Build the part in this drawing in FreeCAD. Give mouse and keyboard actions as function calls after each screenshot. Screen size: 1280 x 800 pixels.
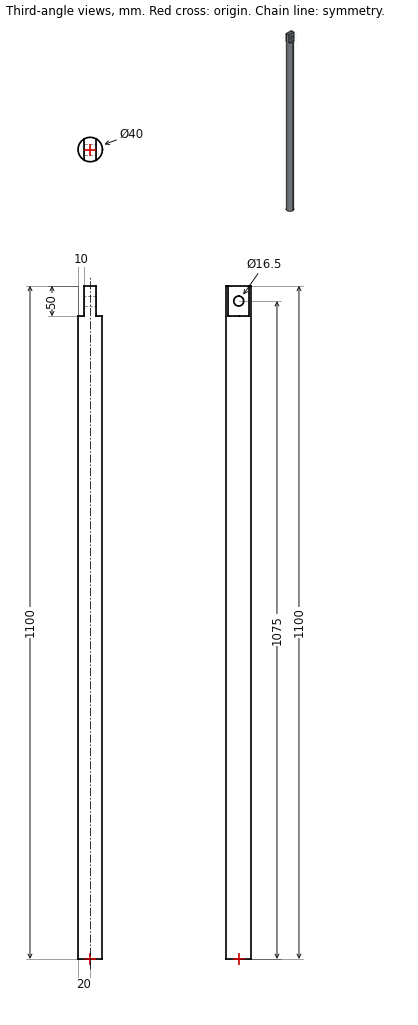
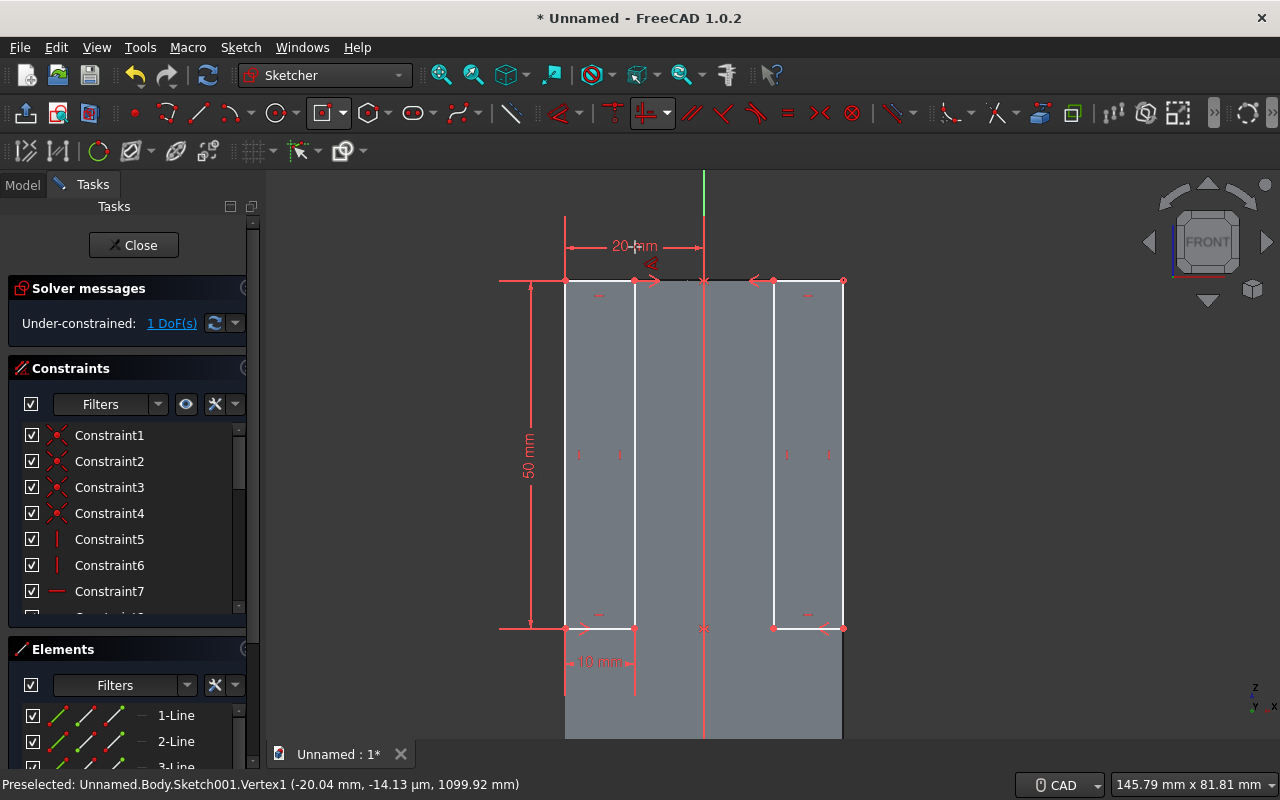
click(565, 281)
click(531, 496)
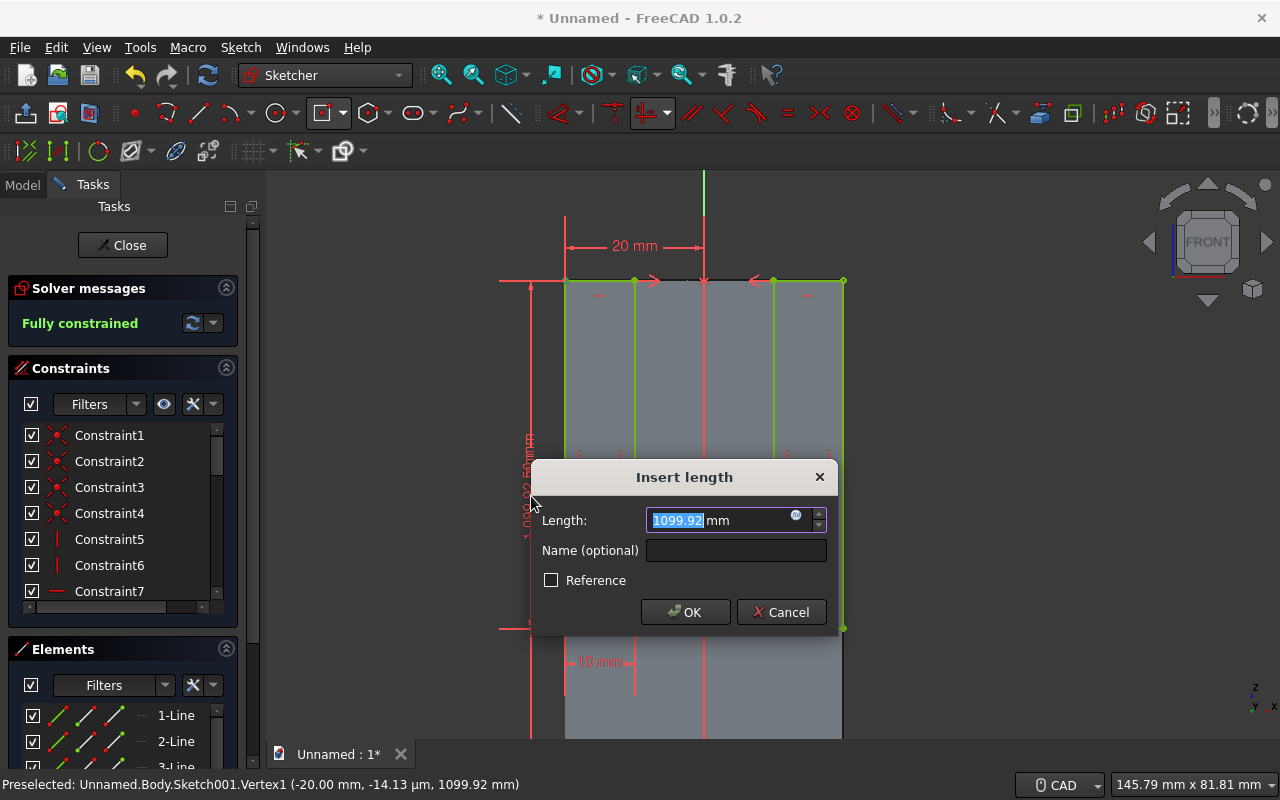
text(1100)
key(Return)
key(Escape)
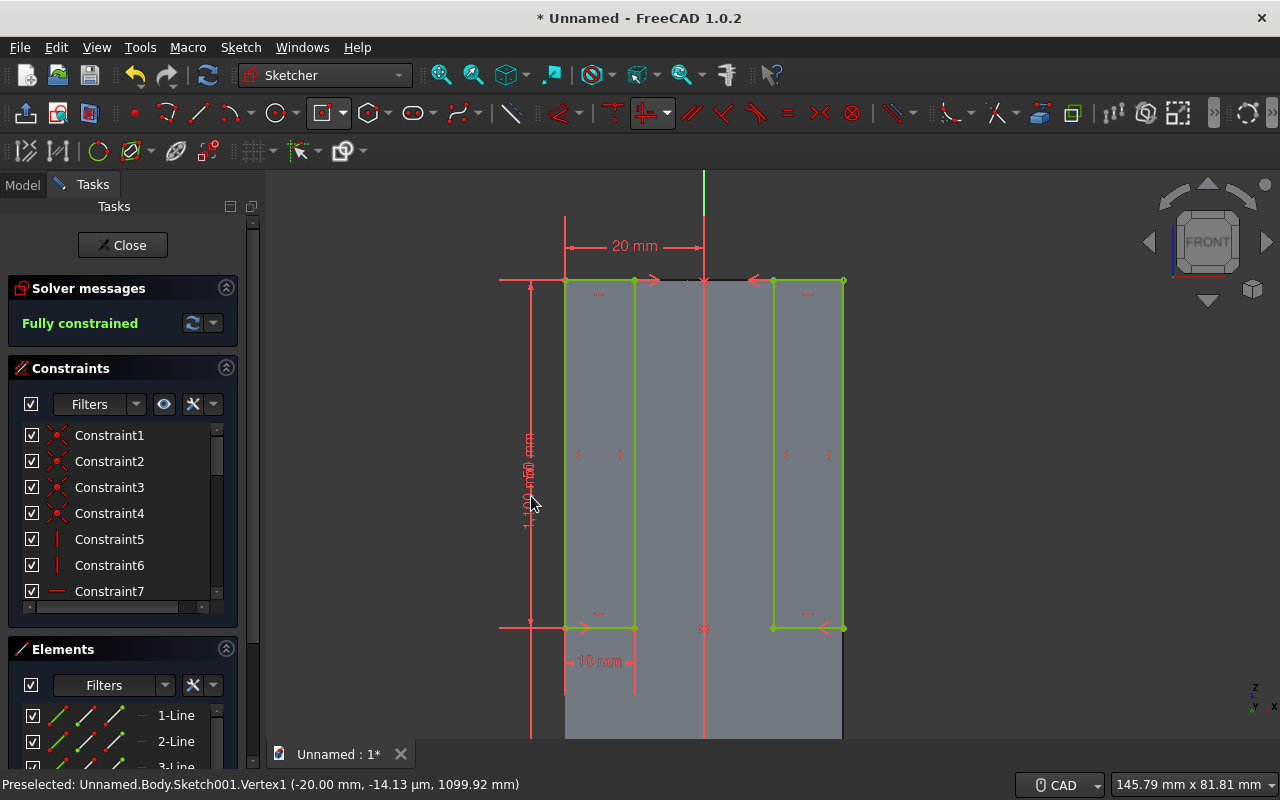
click(123, 245)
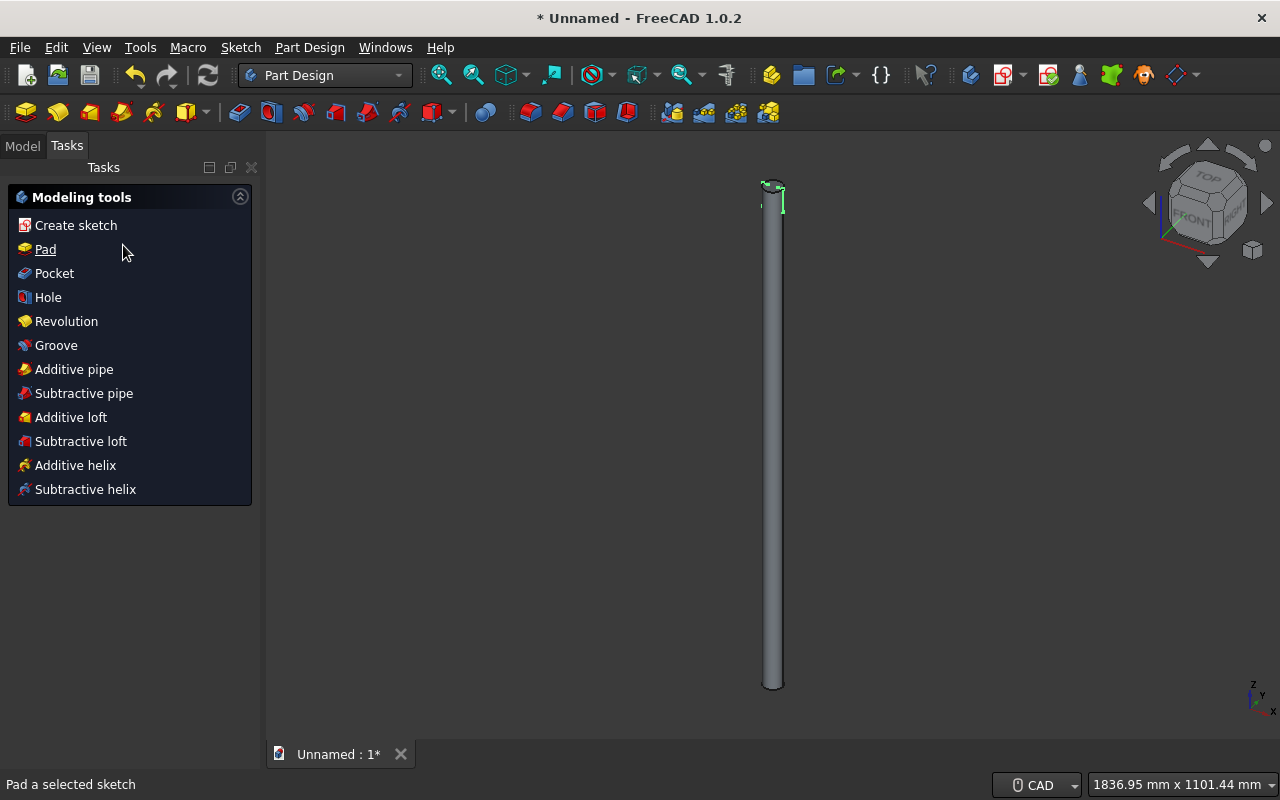
click(240, 112)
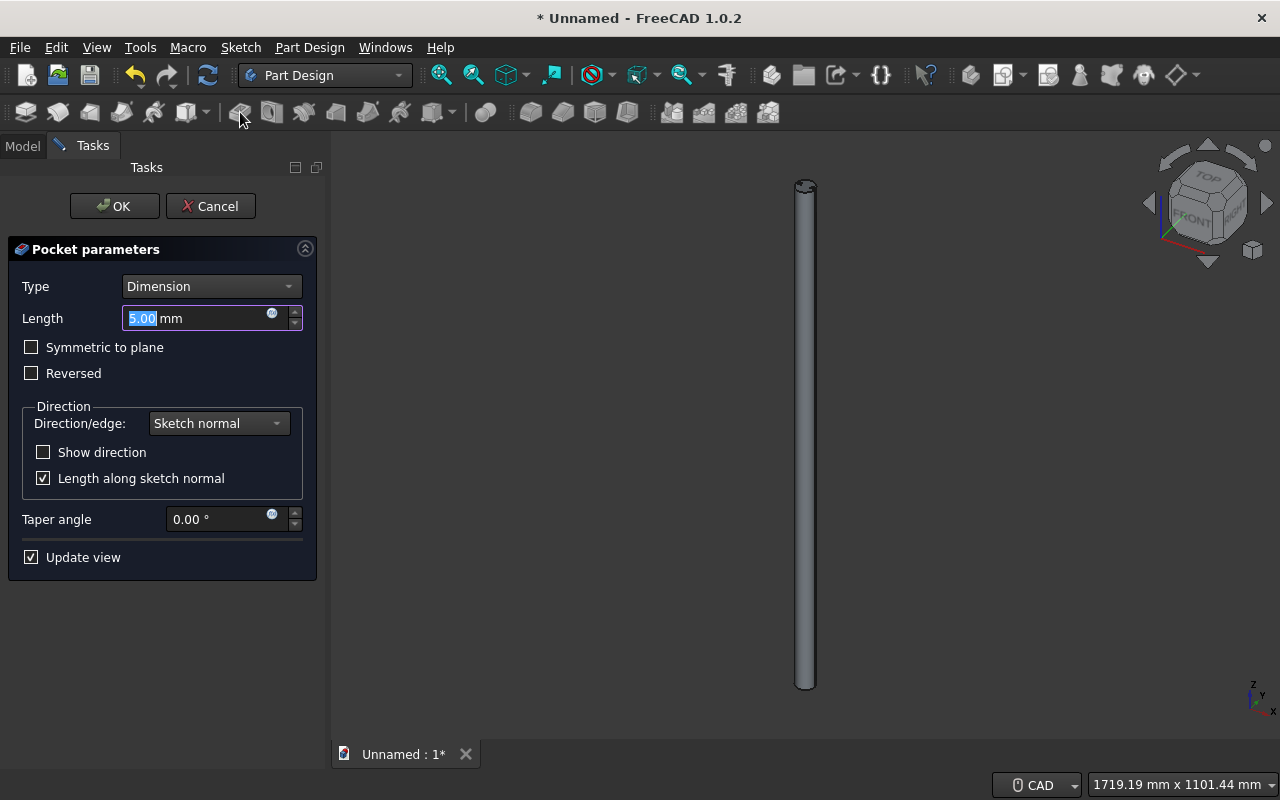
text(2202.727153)
key(Tab)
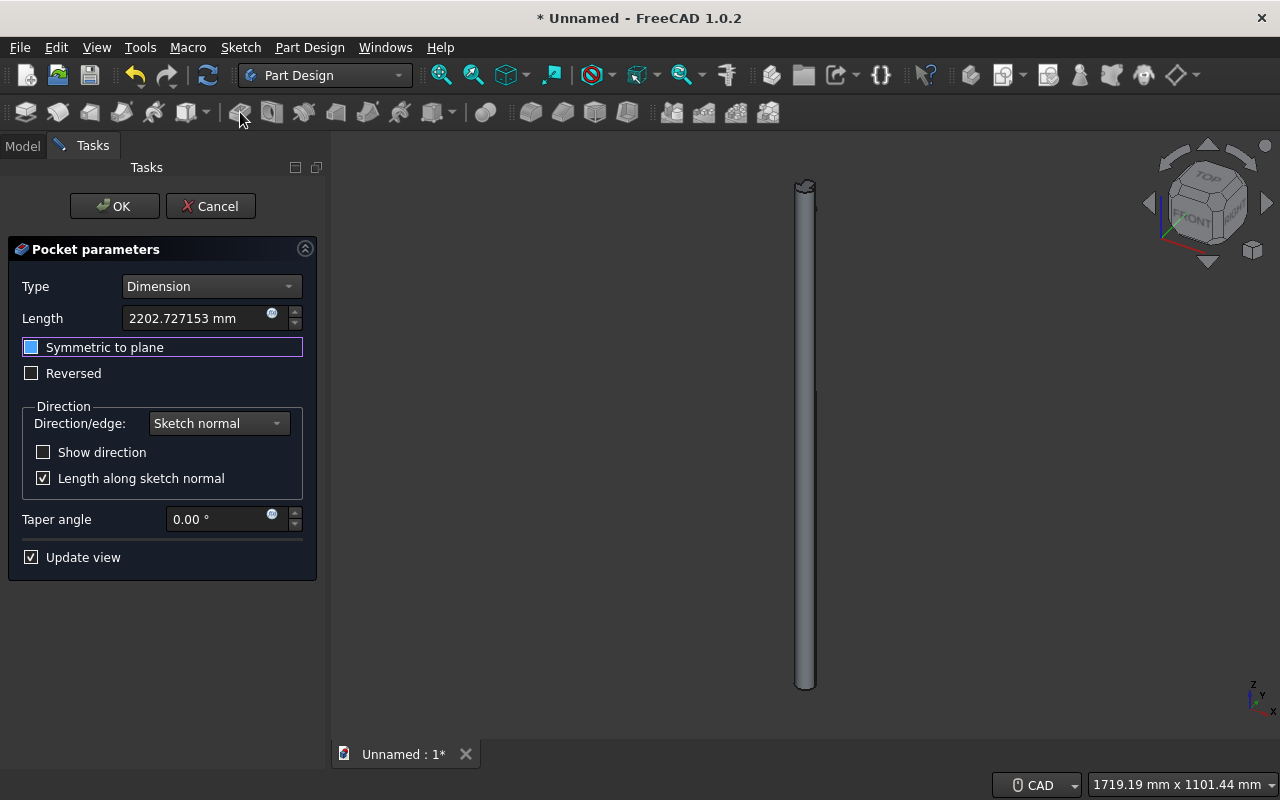
click(30, 347)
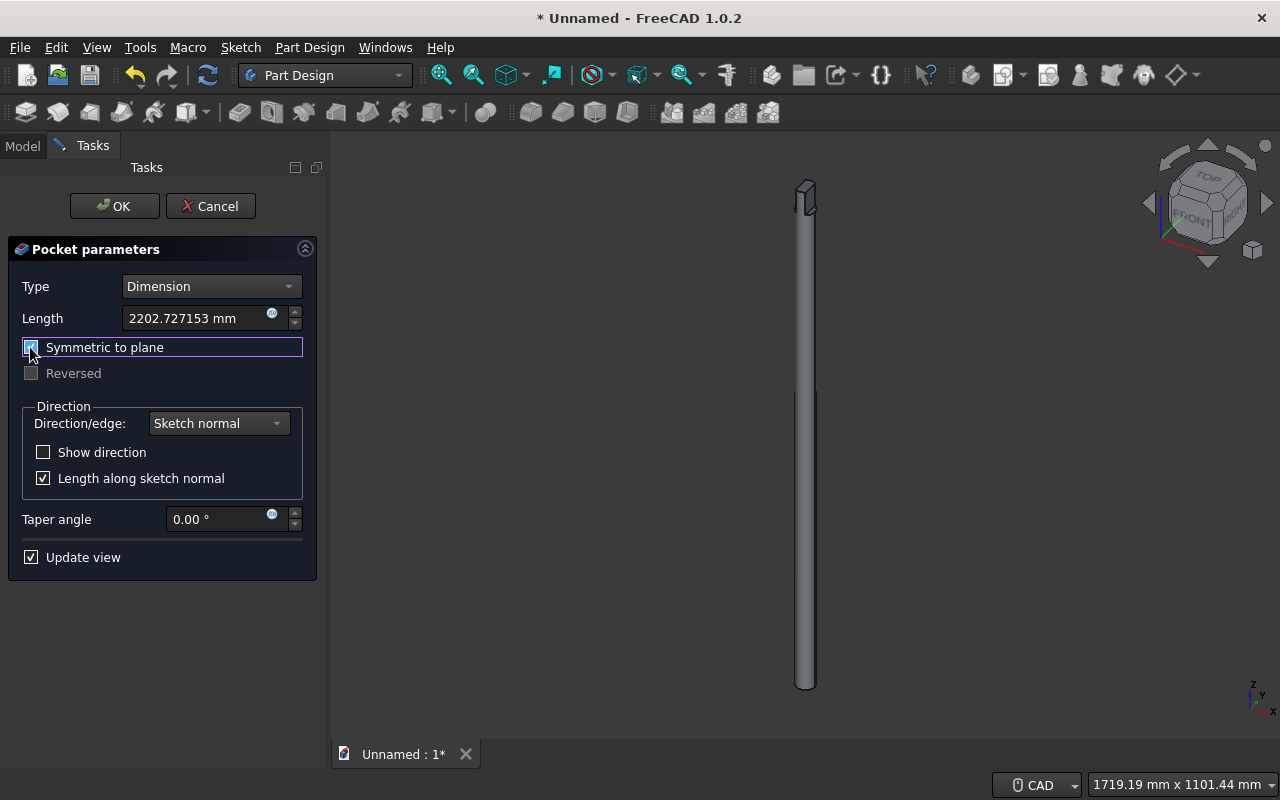
click(115, 206)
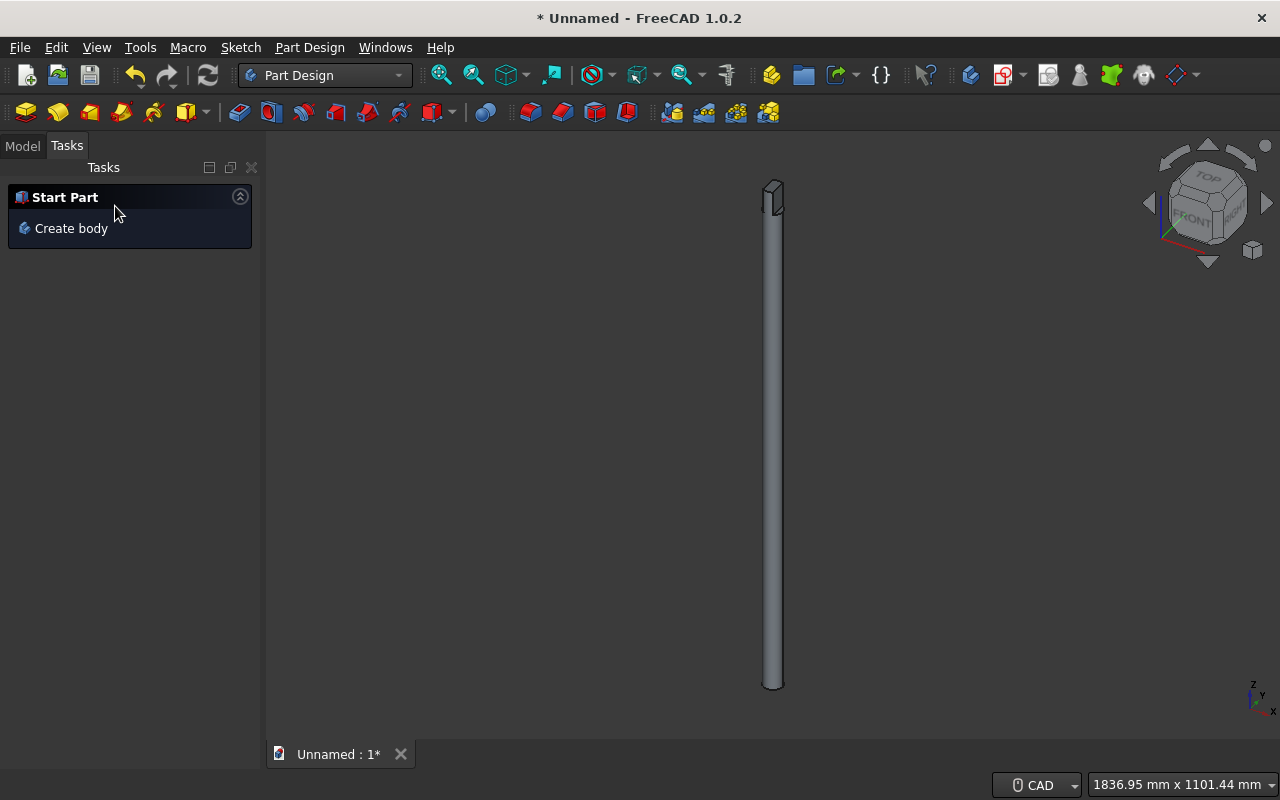
key(6)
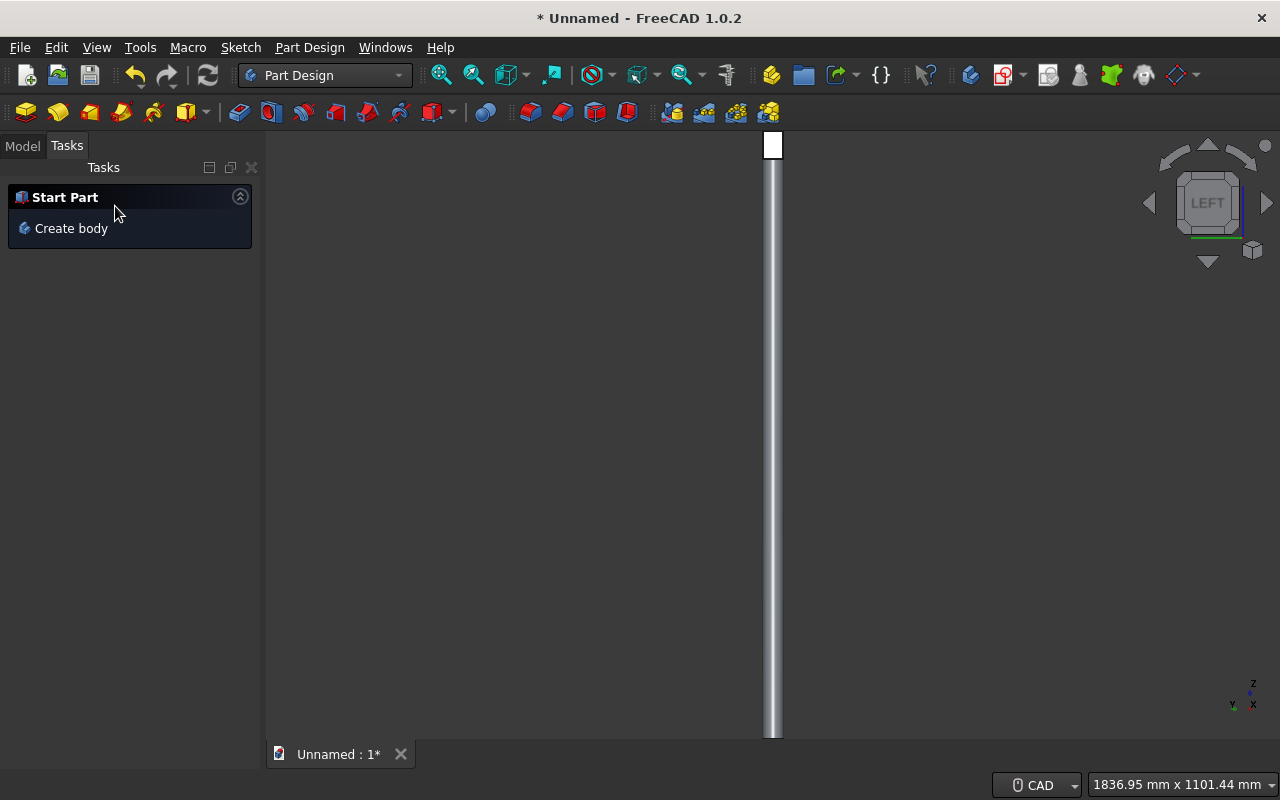
click(442, 76)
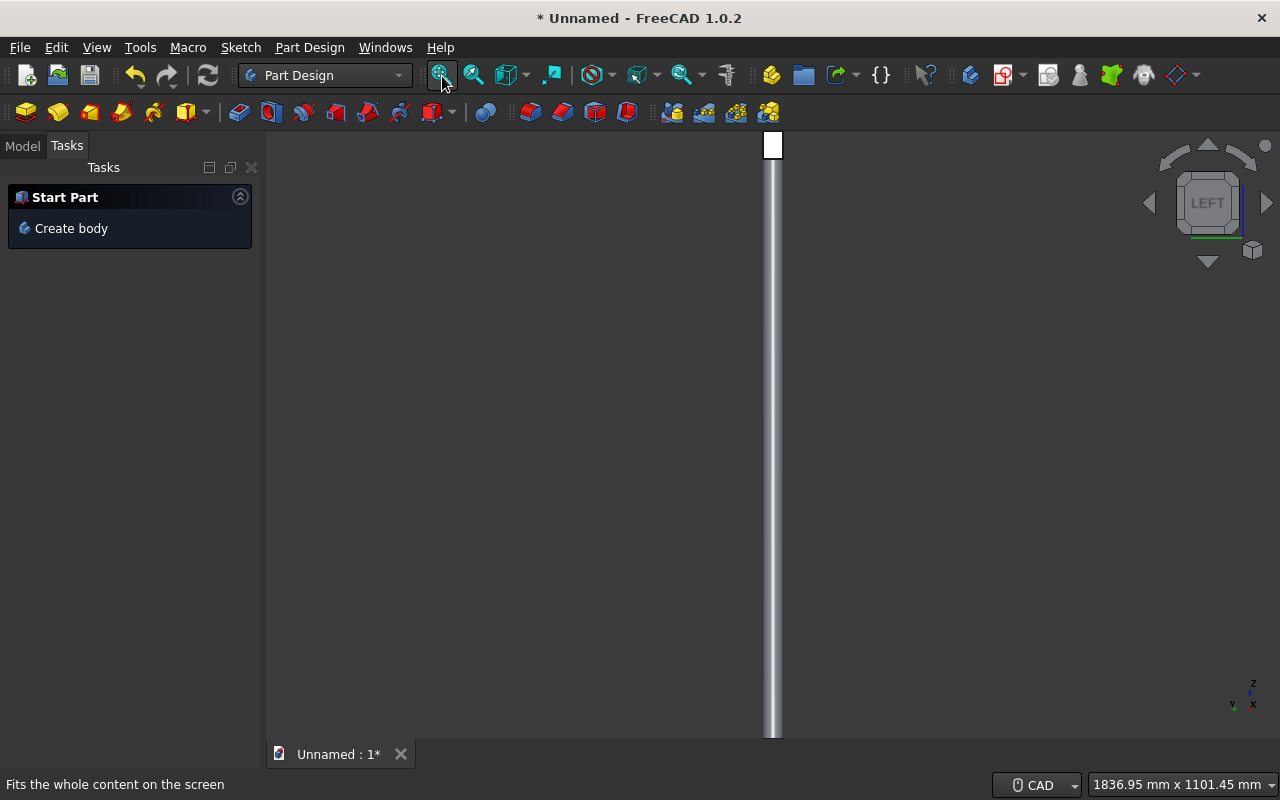
key(2)